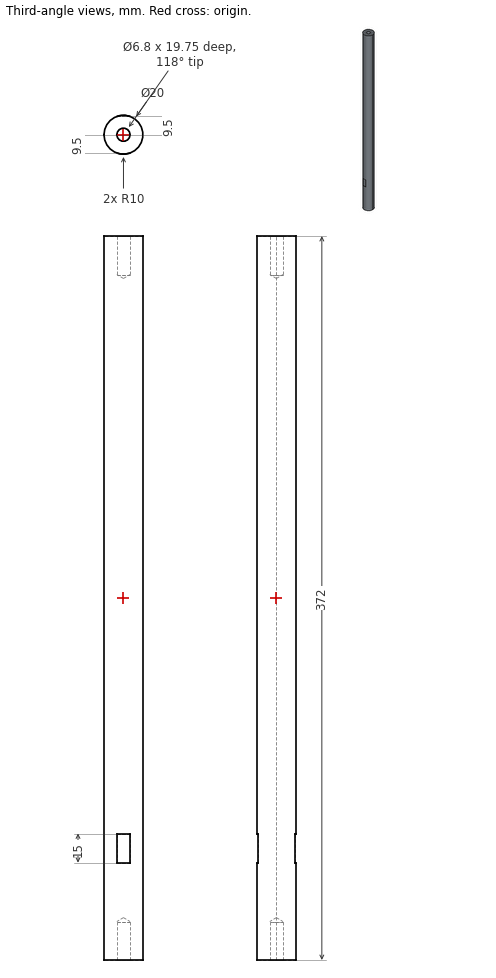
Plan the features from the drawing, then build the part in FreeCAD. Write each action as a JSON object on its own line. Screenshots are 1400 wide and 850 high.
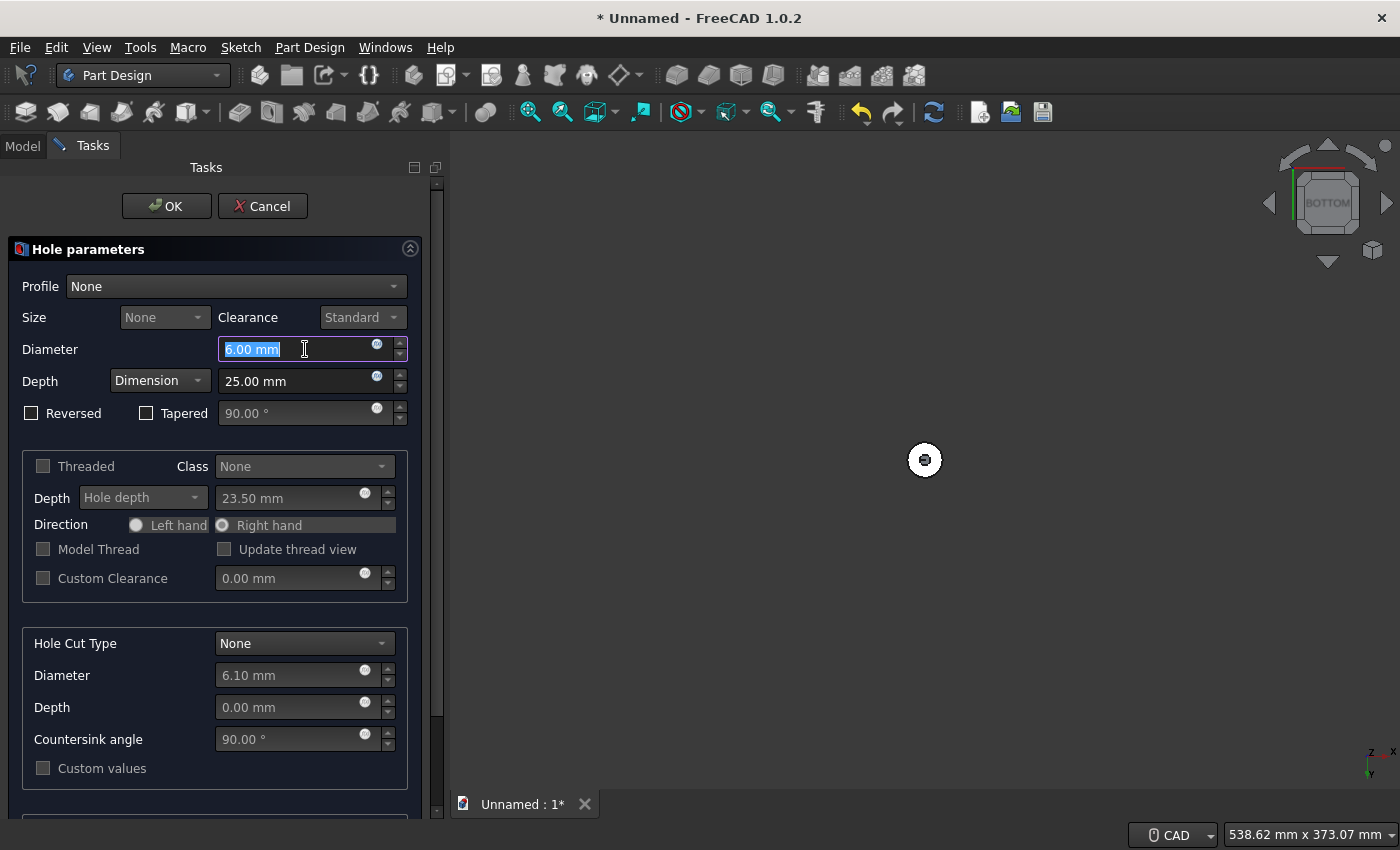
{"action": "type", "text": "6.8"}
{"action": "key", "text": "Tab"}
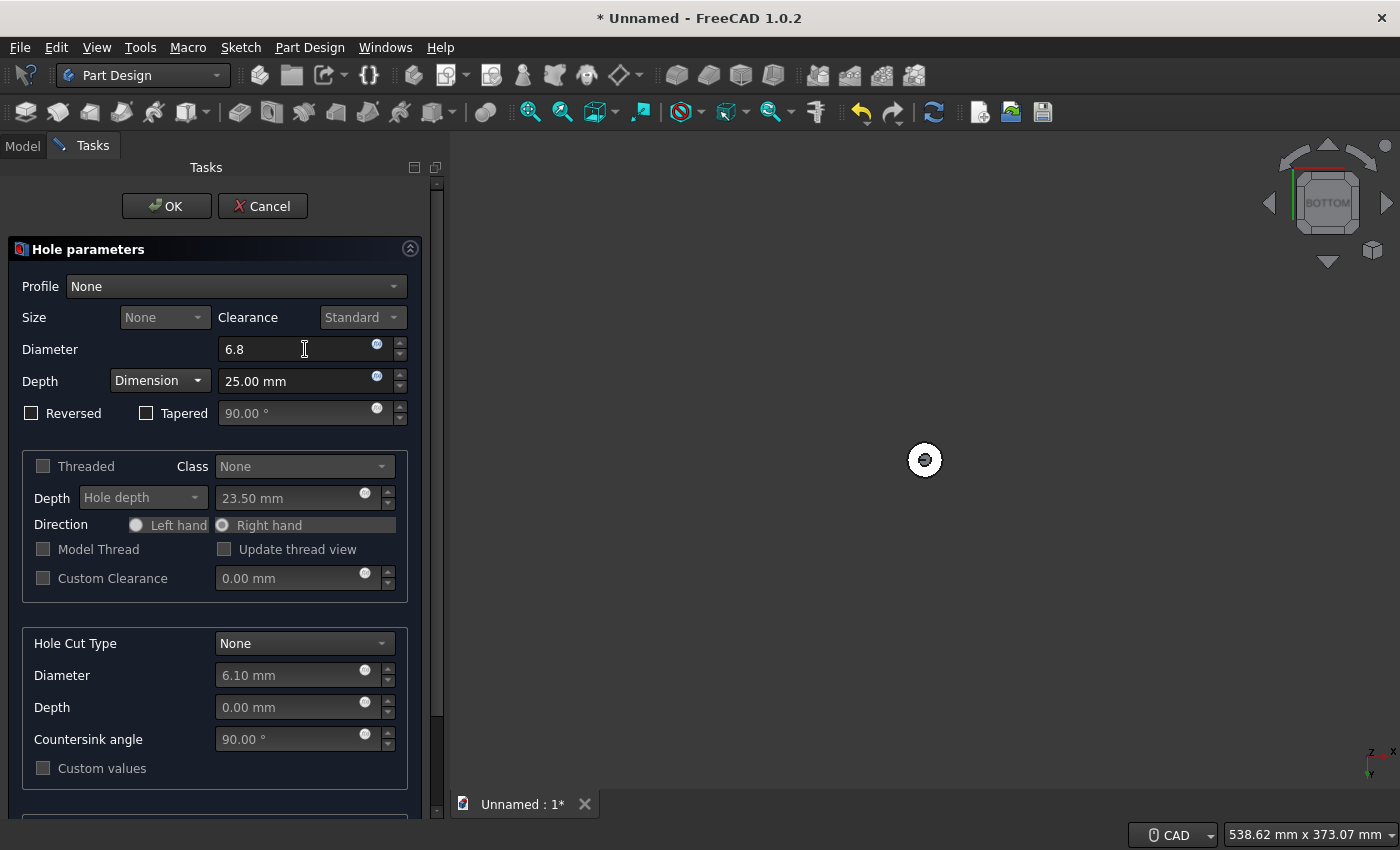
{"action": "triple_click", "coordinate": [305, 381]}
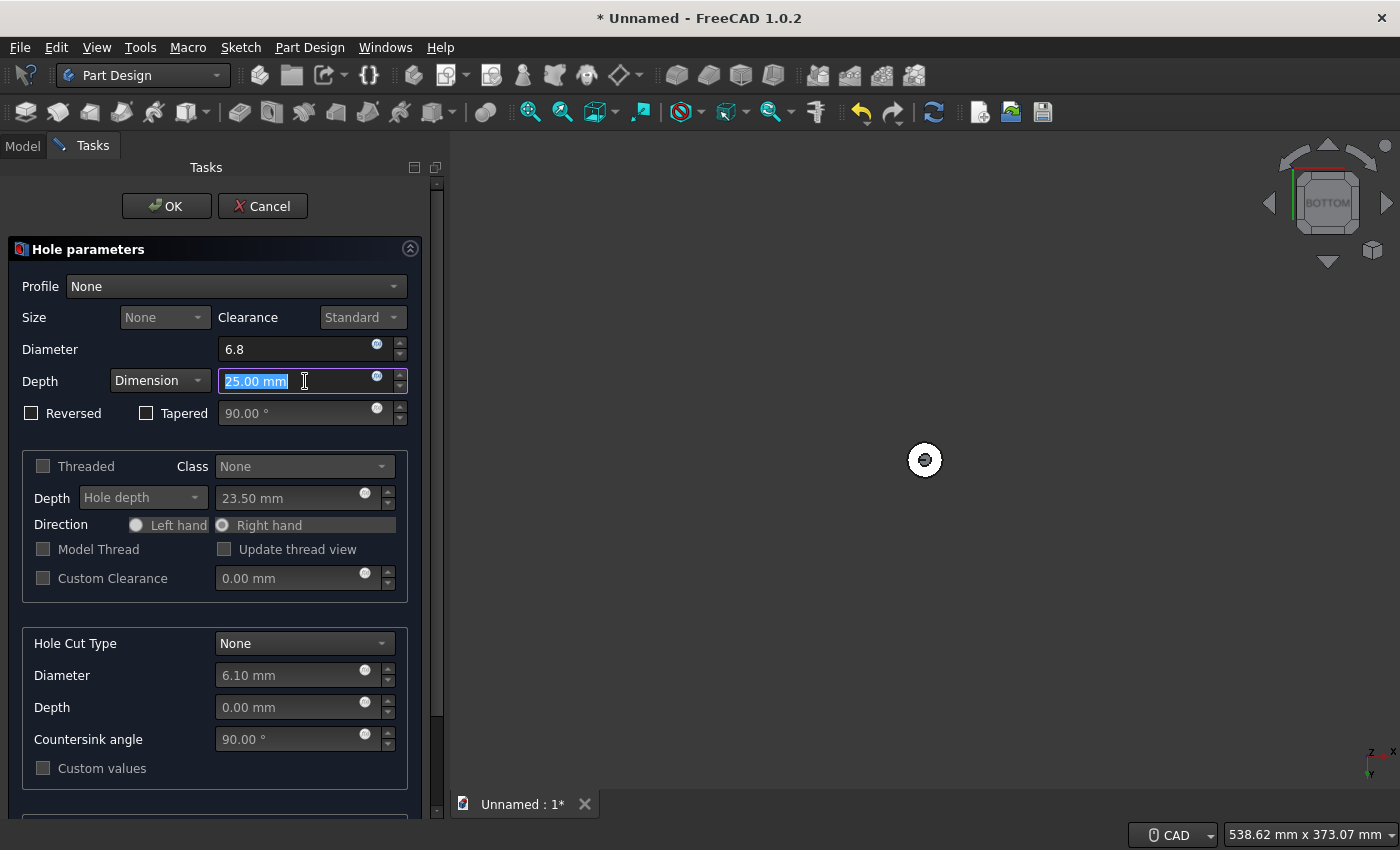
{"action": "type", "text": "19.75"}
{"action": "key", "text": "Tab"}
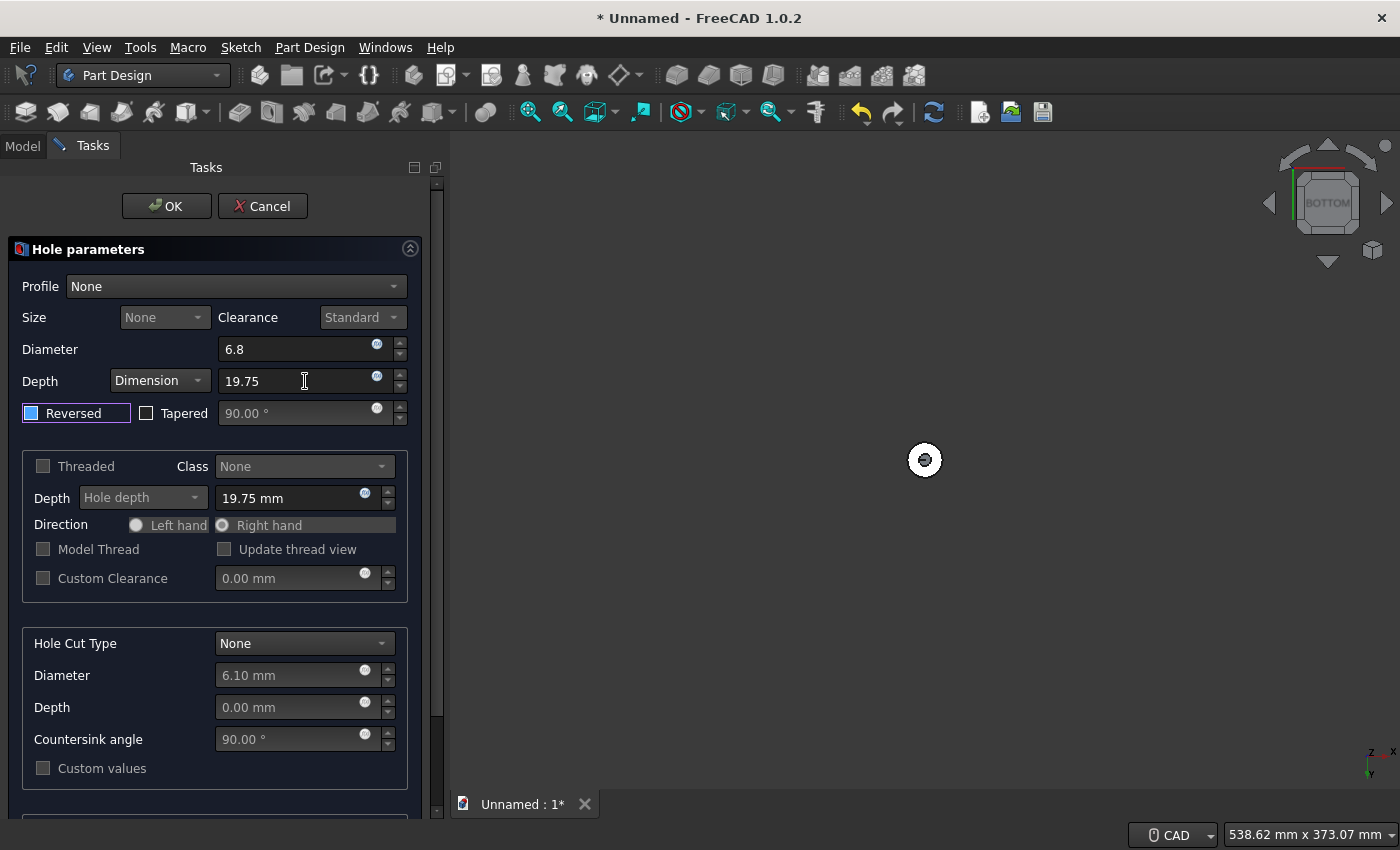
{"action": "left_click", "coordinate": [167, 206]}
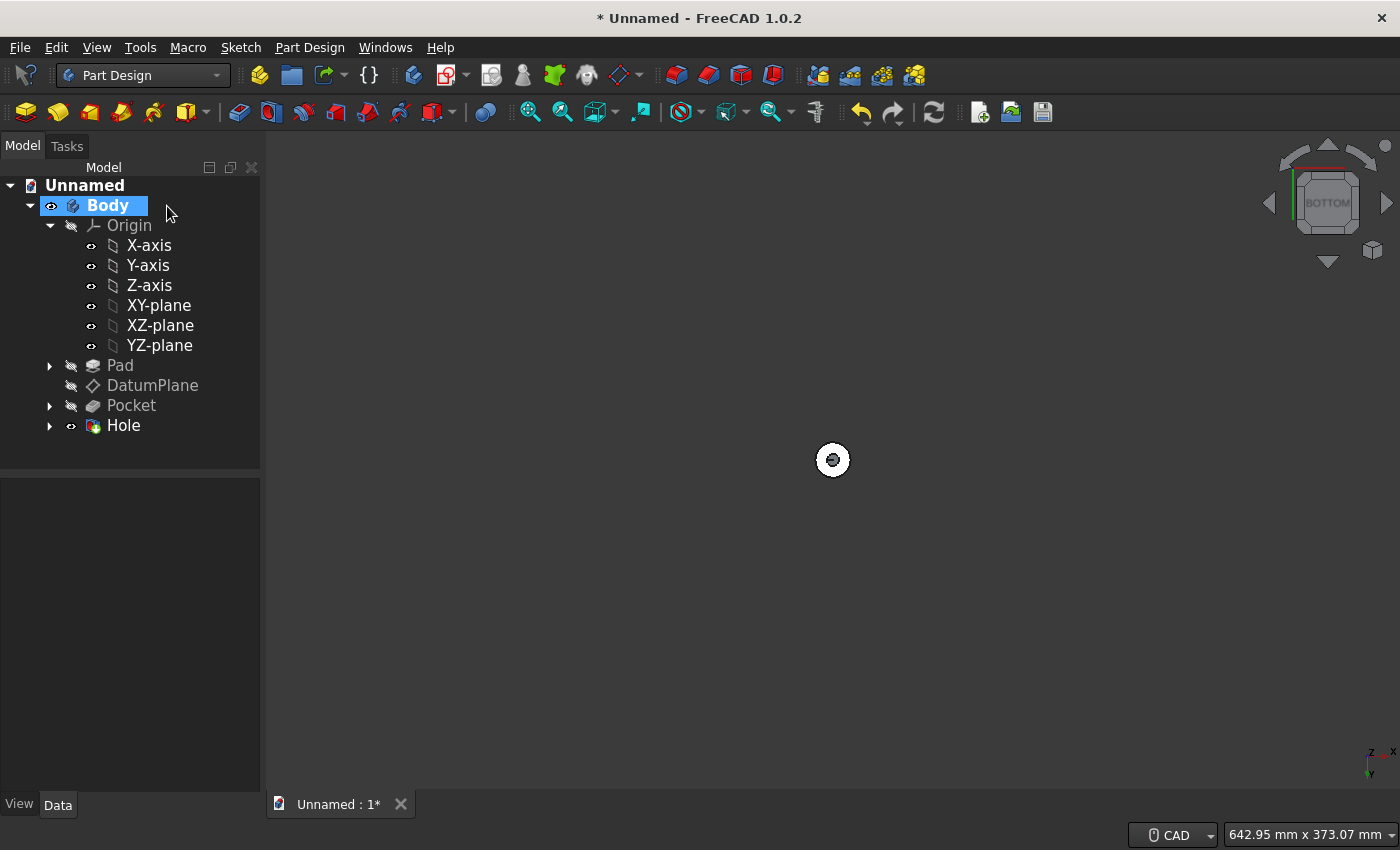
{"action": "left_click", "coordinate": [532, 112]}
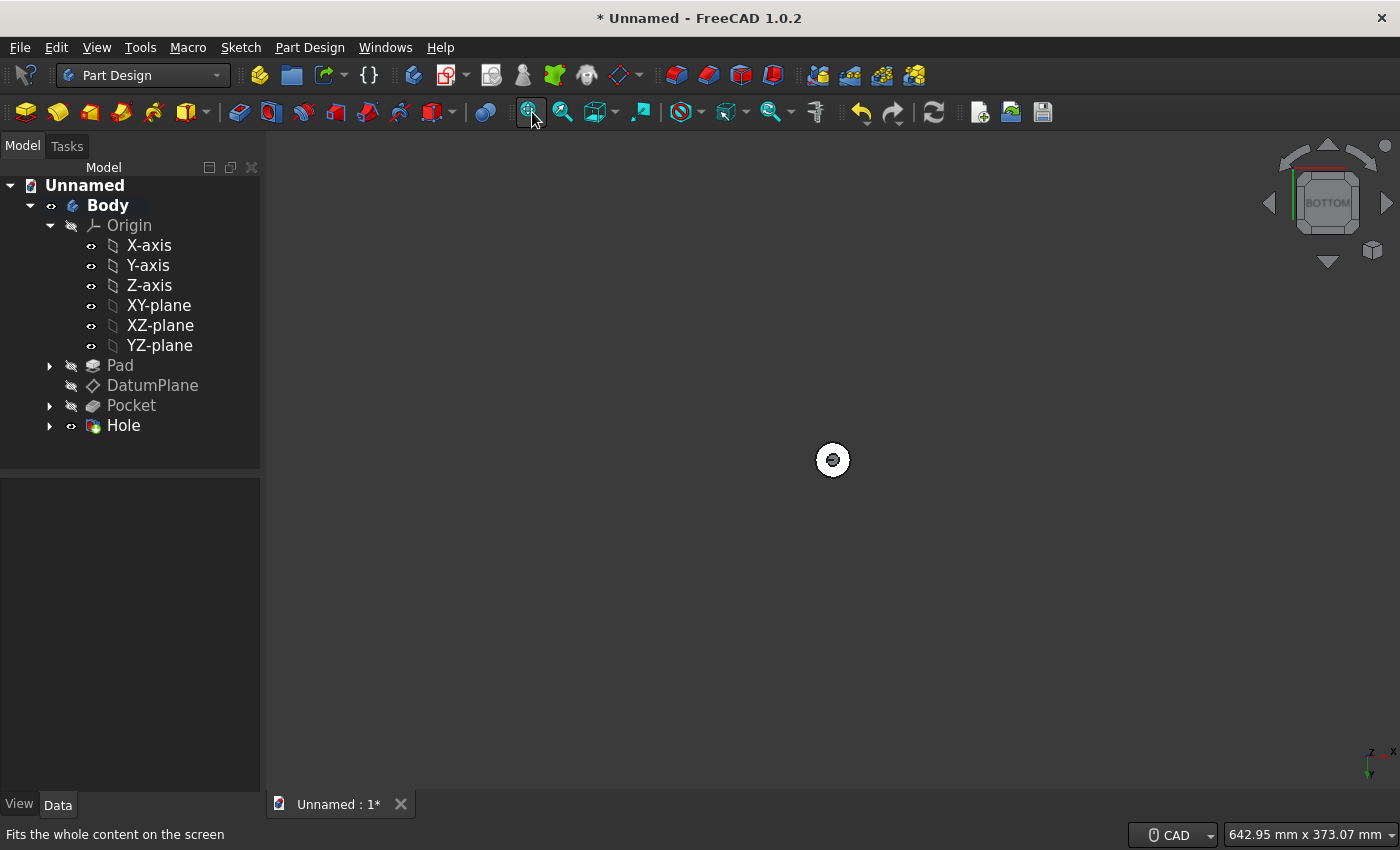
{"action": "key", "text": "0"}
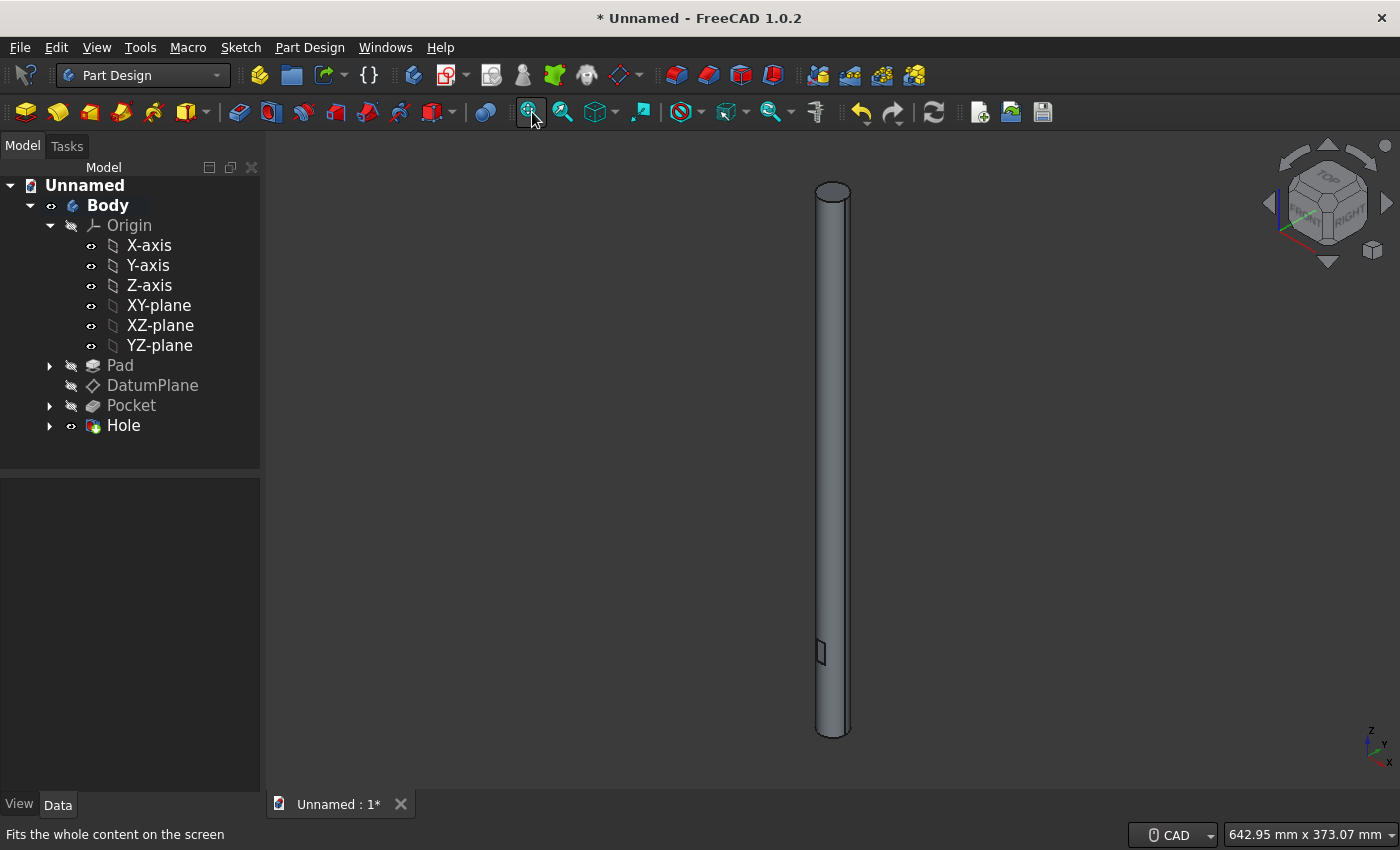
{"action": "left_click", "coordinate": [833, 191]}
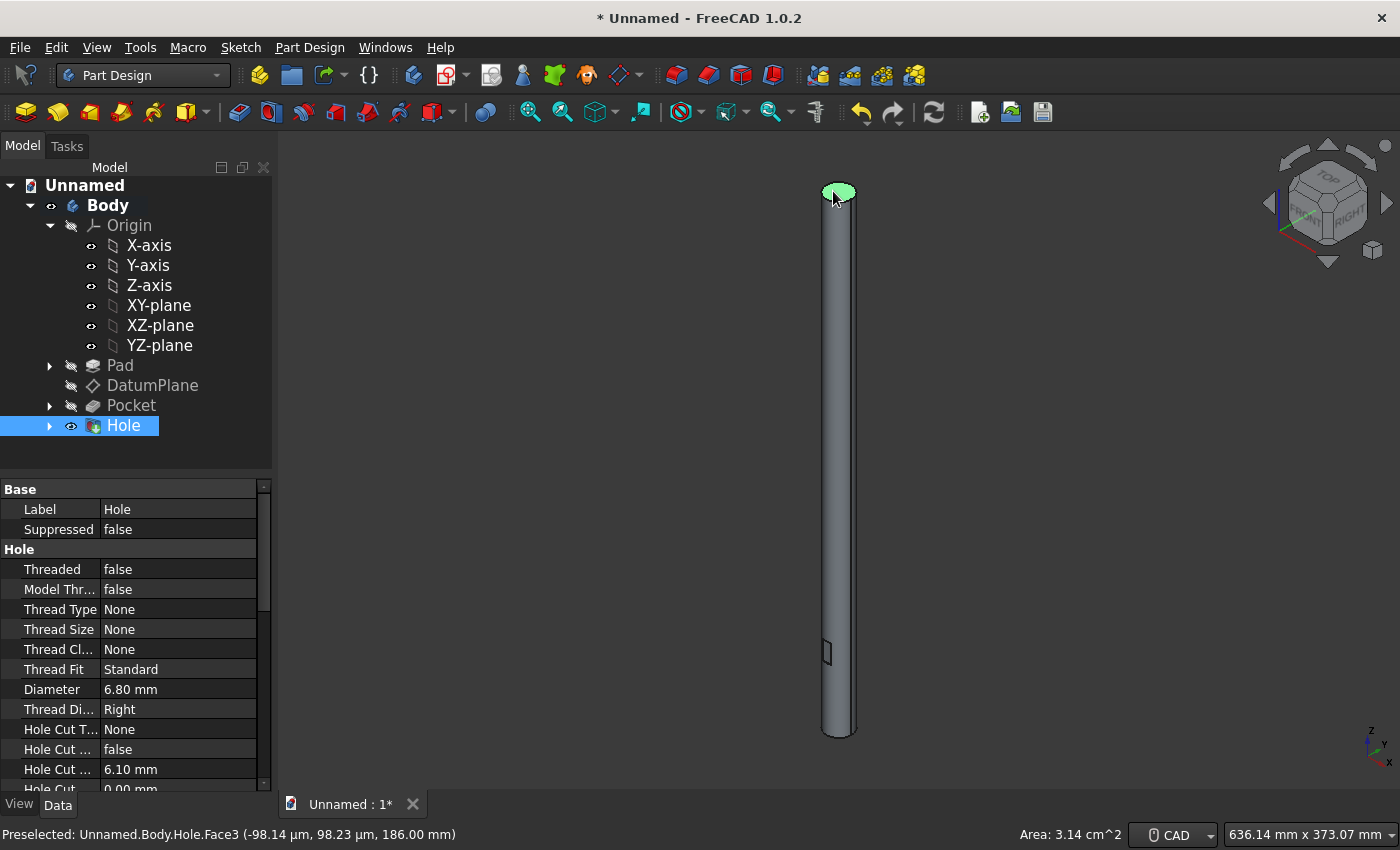
{"action": "left_click", "coordinate": [446, 76]}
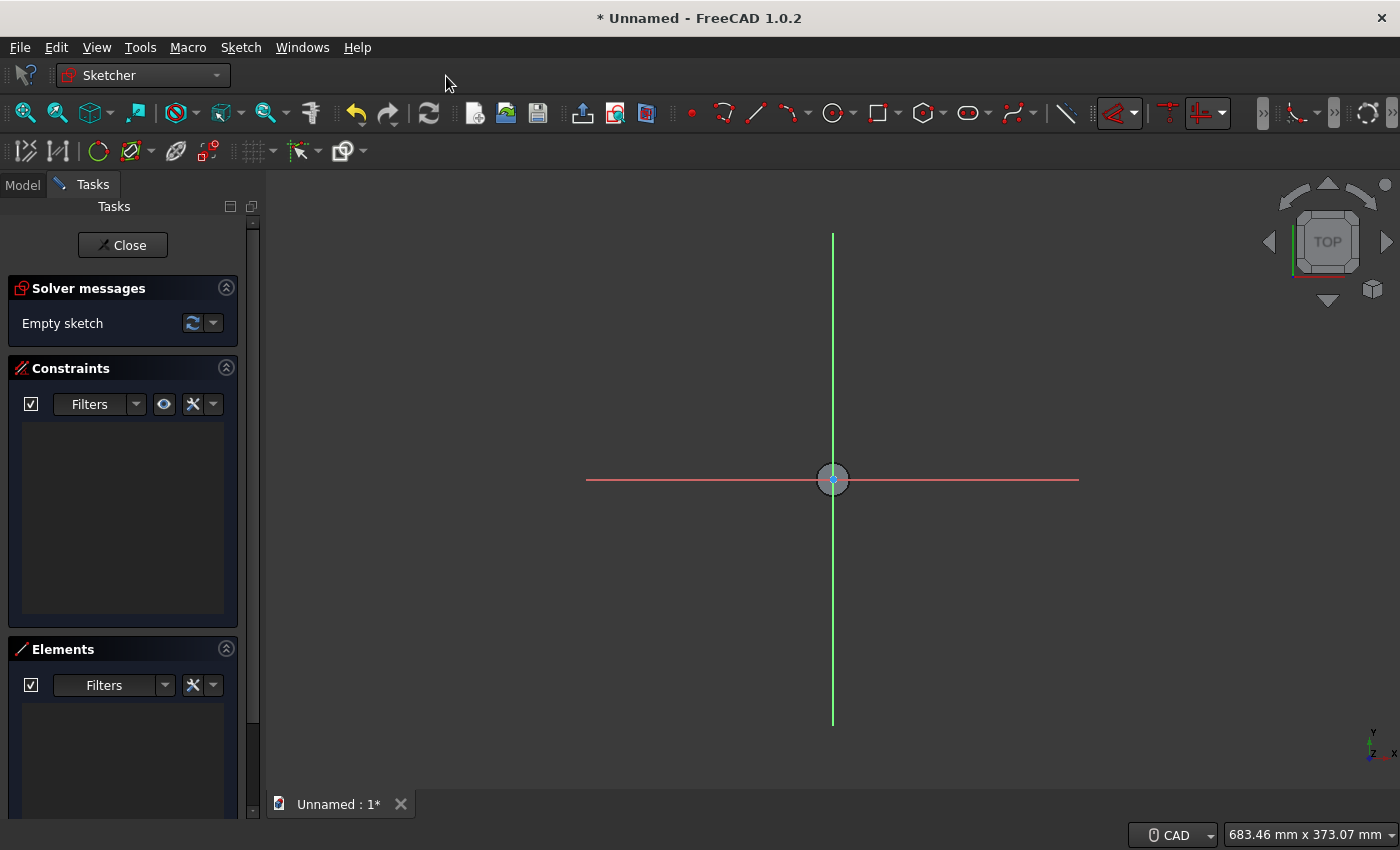
{"action": "scroll", "coordinate": [837, 479], "scroll_direction": "up", "scroll_amount": 15}